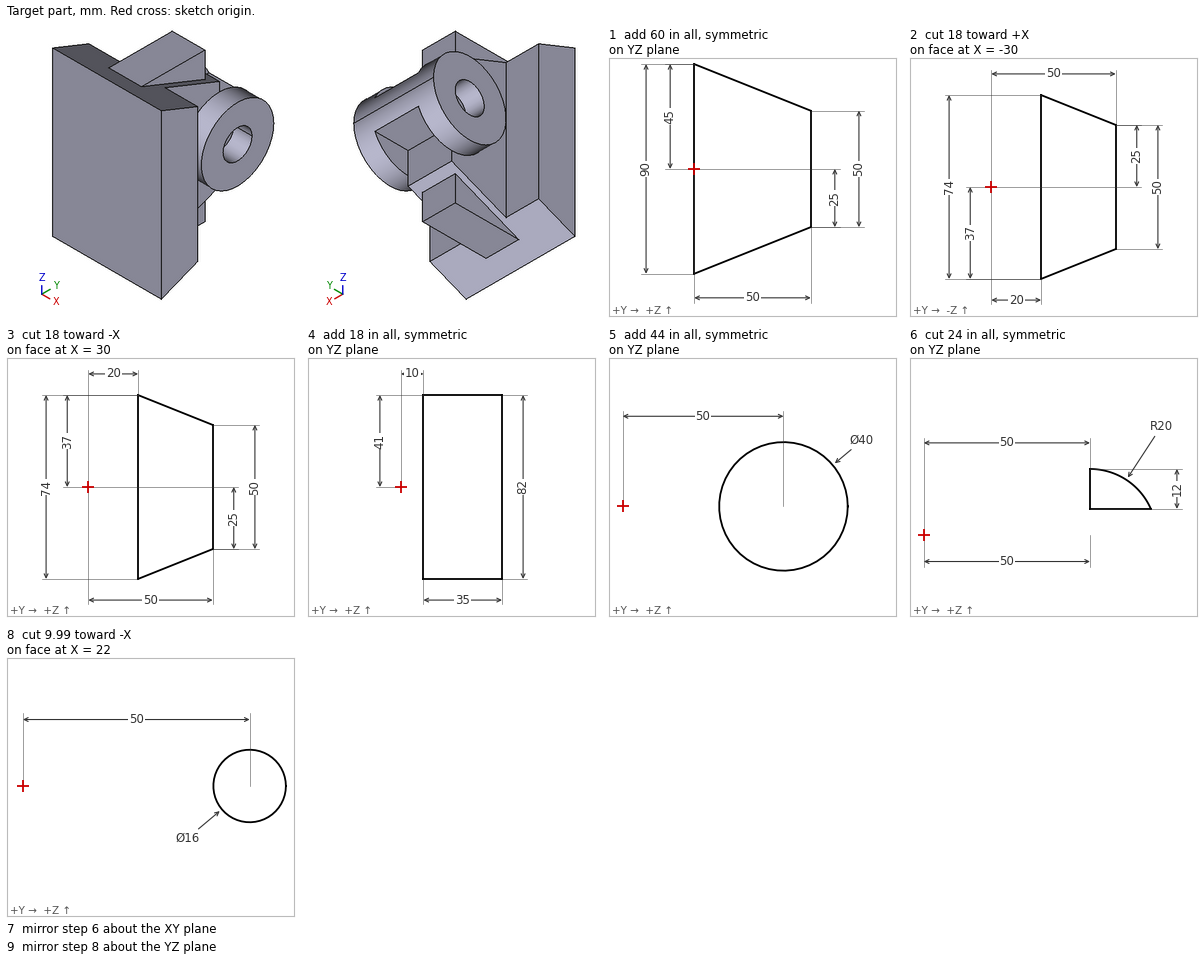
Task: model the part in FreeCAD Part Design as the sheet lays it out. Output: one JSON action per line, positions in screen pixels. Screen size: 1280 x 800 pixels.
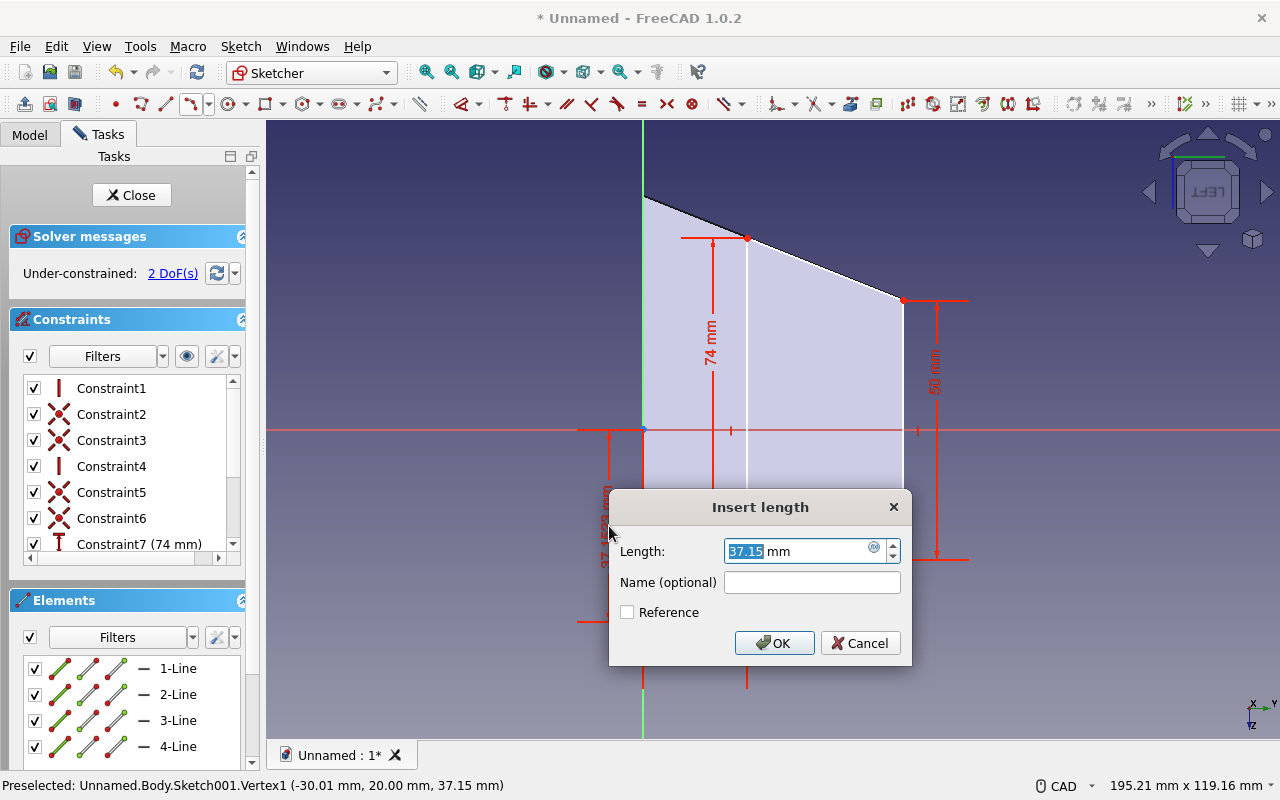
{"action": "type", "text": "37"}
{"action": "key", "text": "Return"}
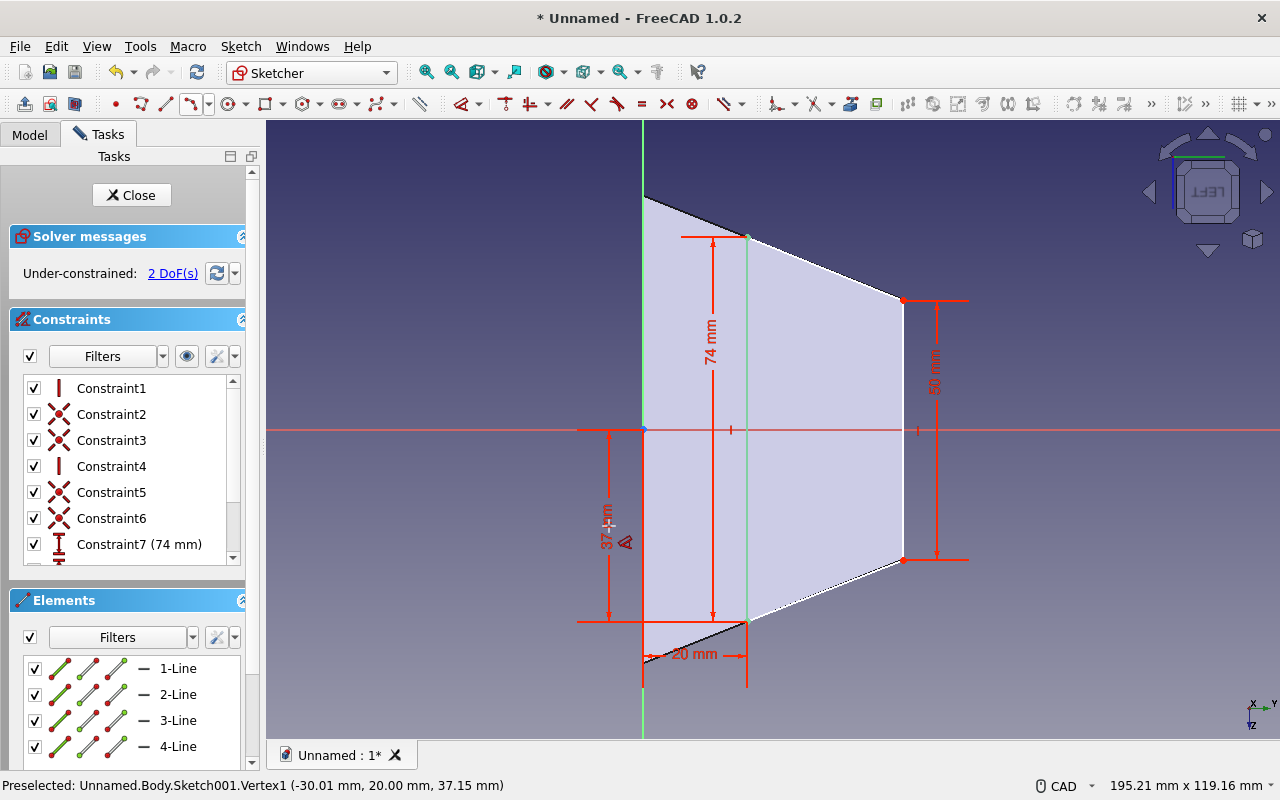
{"action": "left_click", "coordinate": [903, 301]}
{"action": "left_click", "coordinate": [773, 267]}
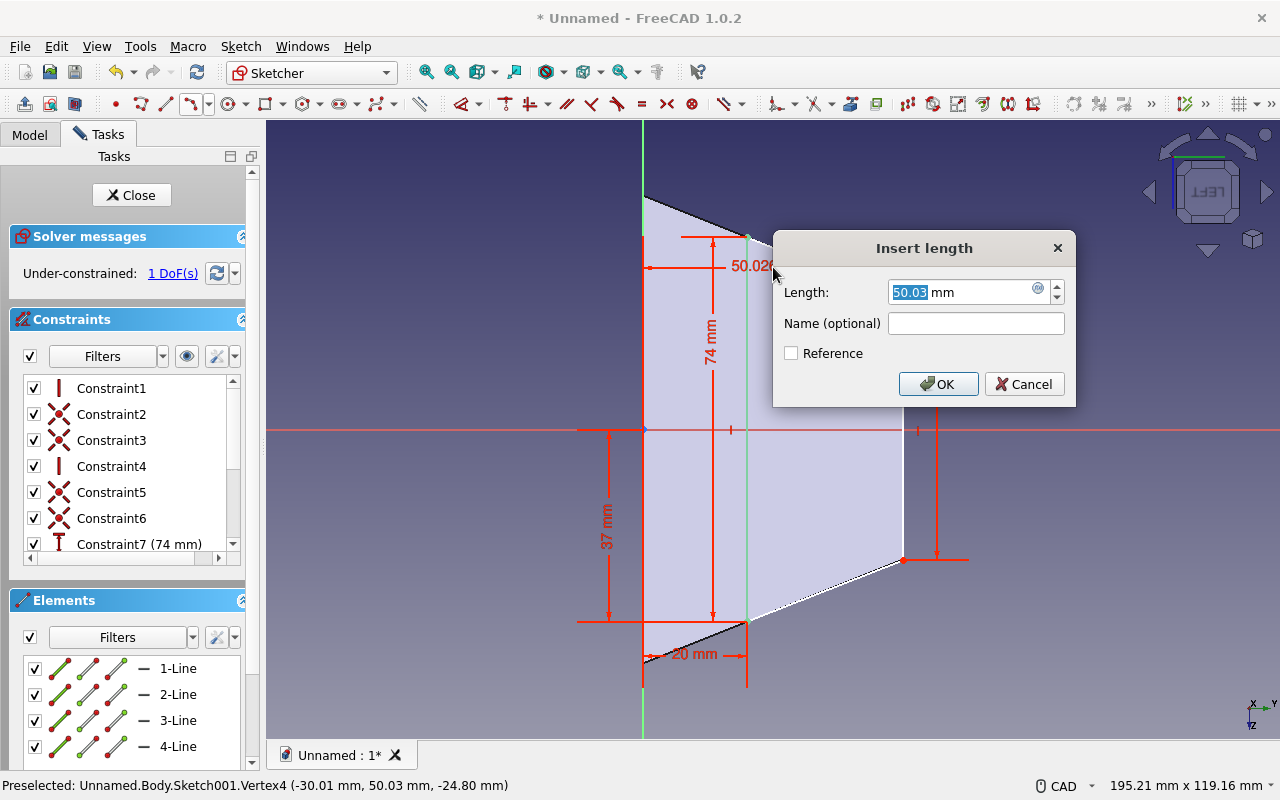
{"action": "type", "text": "50"}
{"action": "key", "text": "Return"}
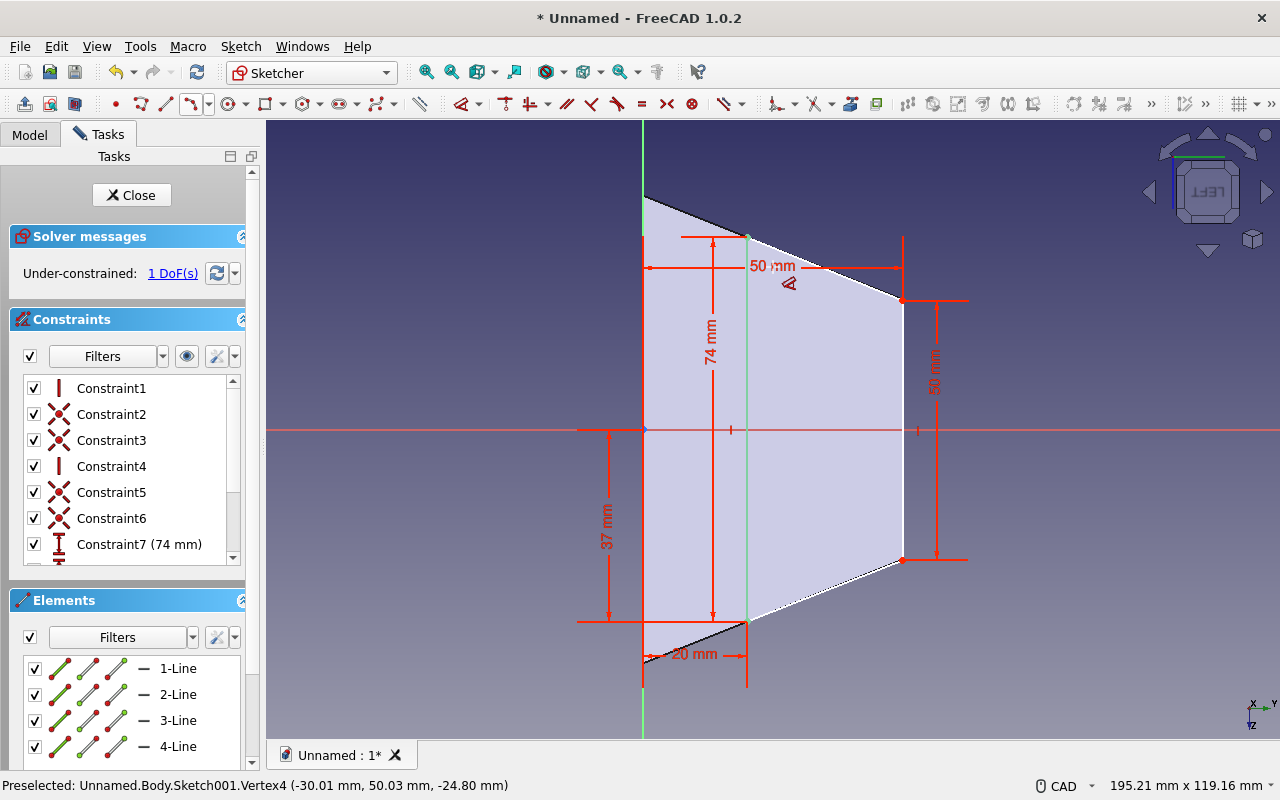
{"action": "left_click", "coordinate": [903, 301]}
{"action": "left_click", "coordinate": [937, 335]}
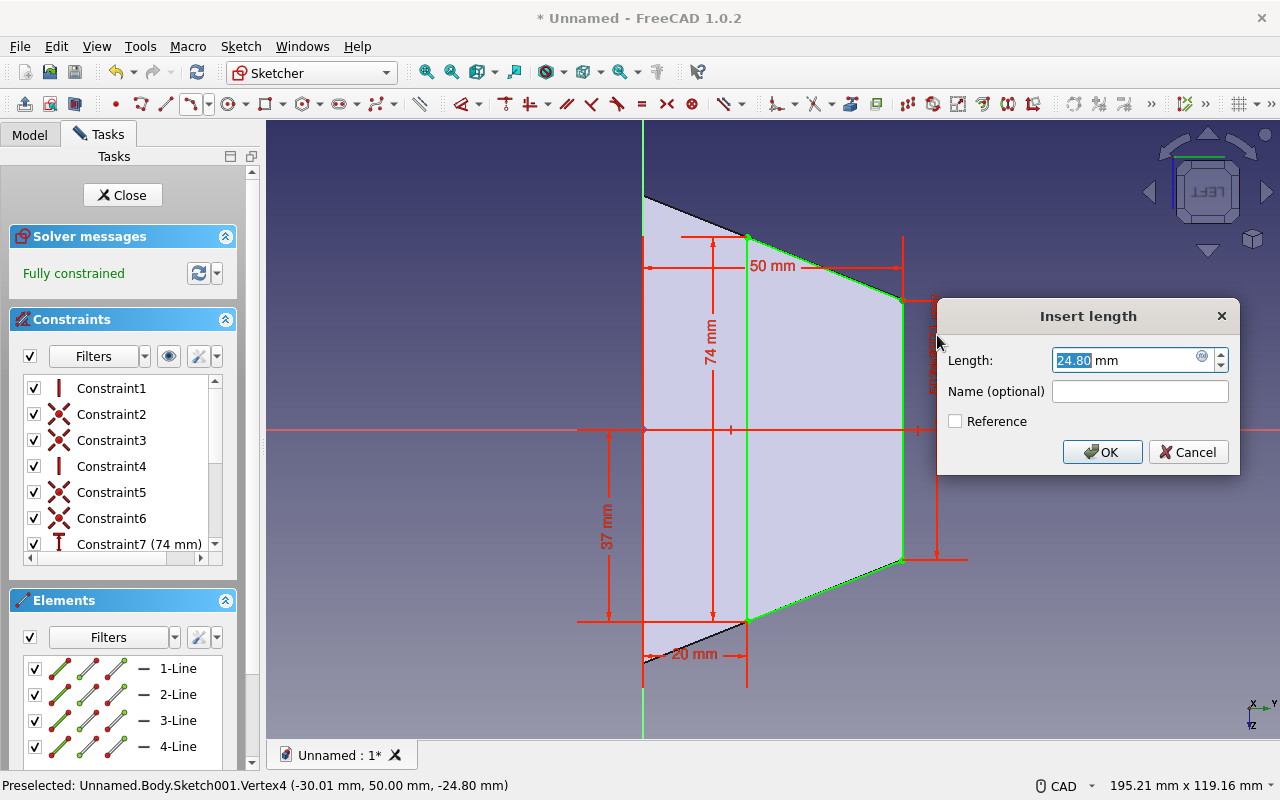
{"action": "type", "text": "25"}
{"action": "key", "text": "Return"}
{"action": "key", "text": "Escape"}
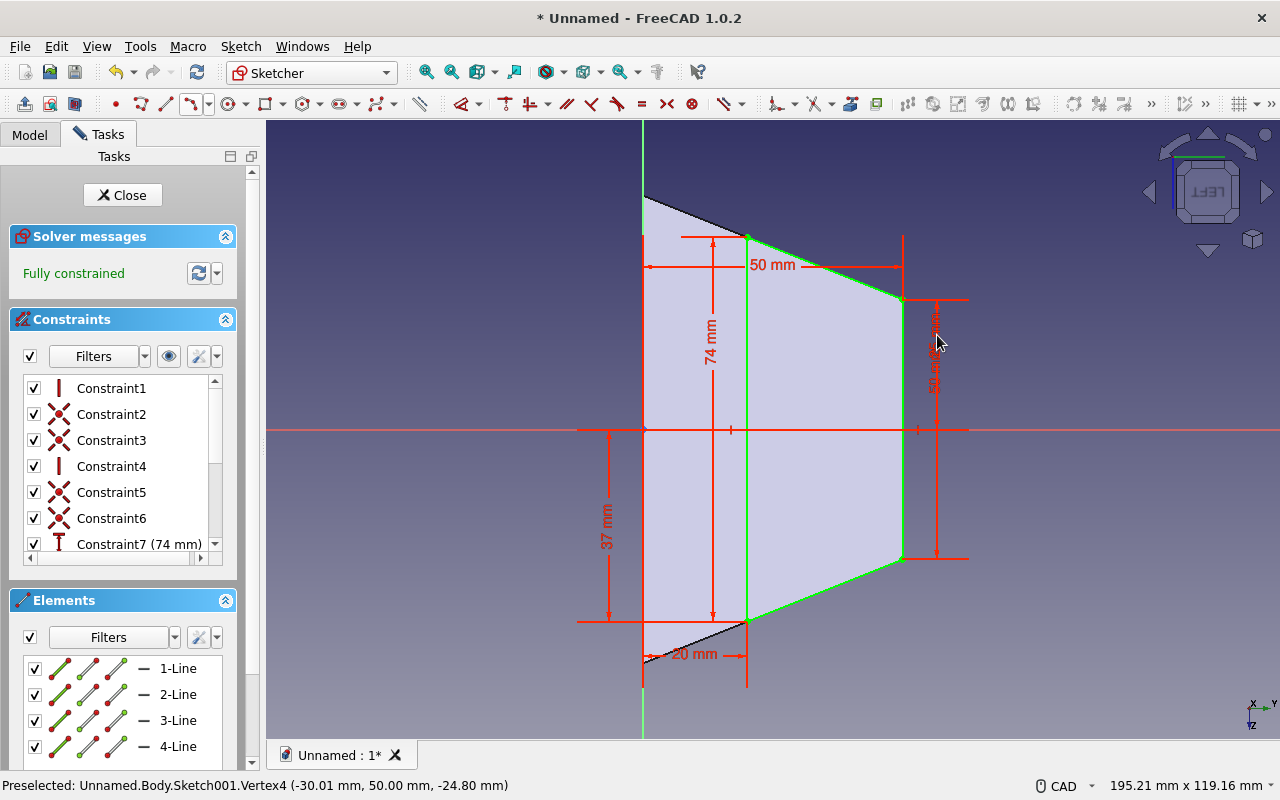
{"action": "left_click", "coordinate": [123, 195]}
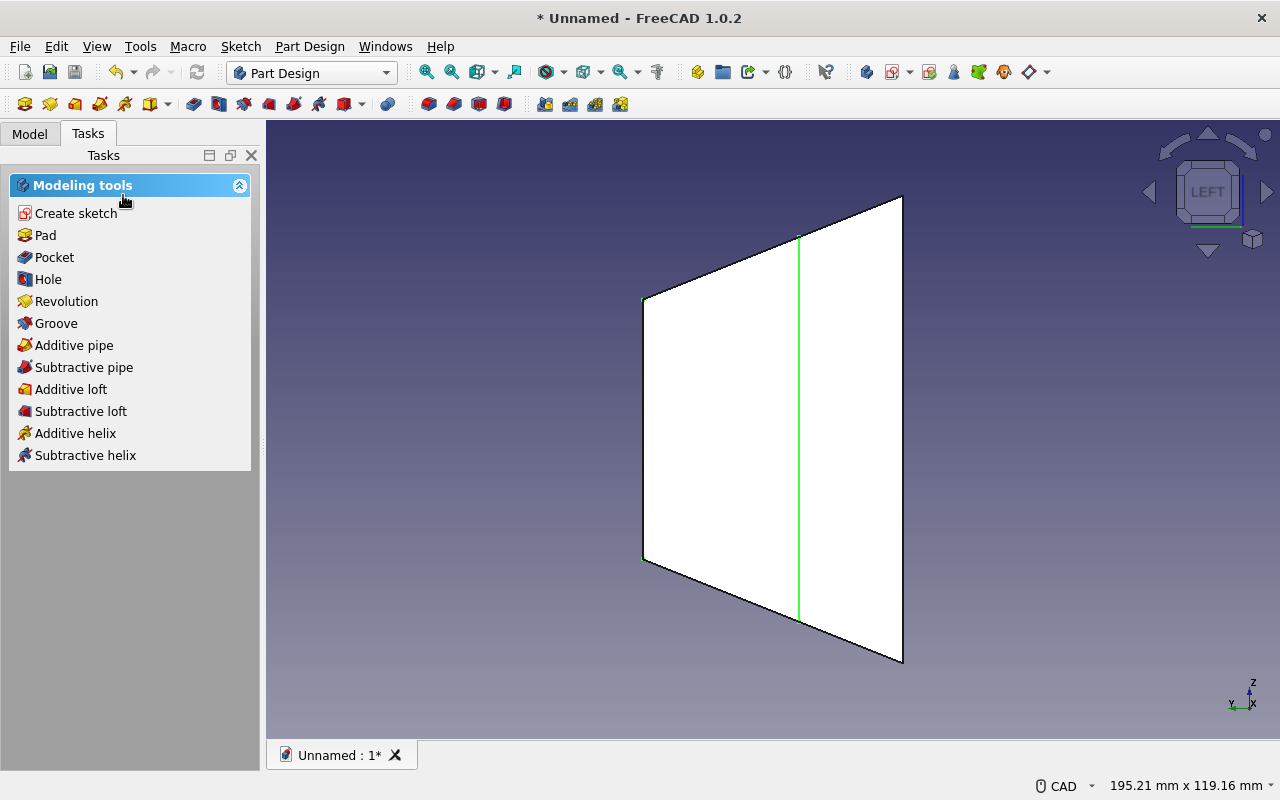
{"action": "left_click", "coordinate": [194, 104]}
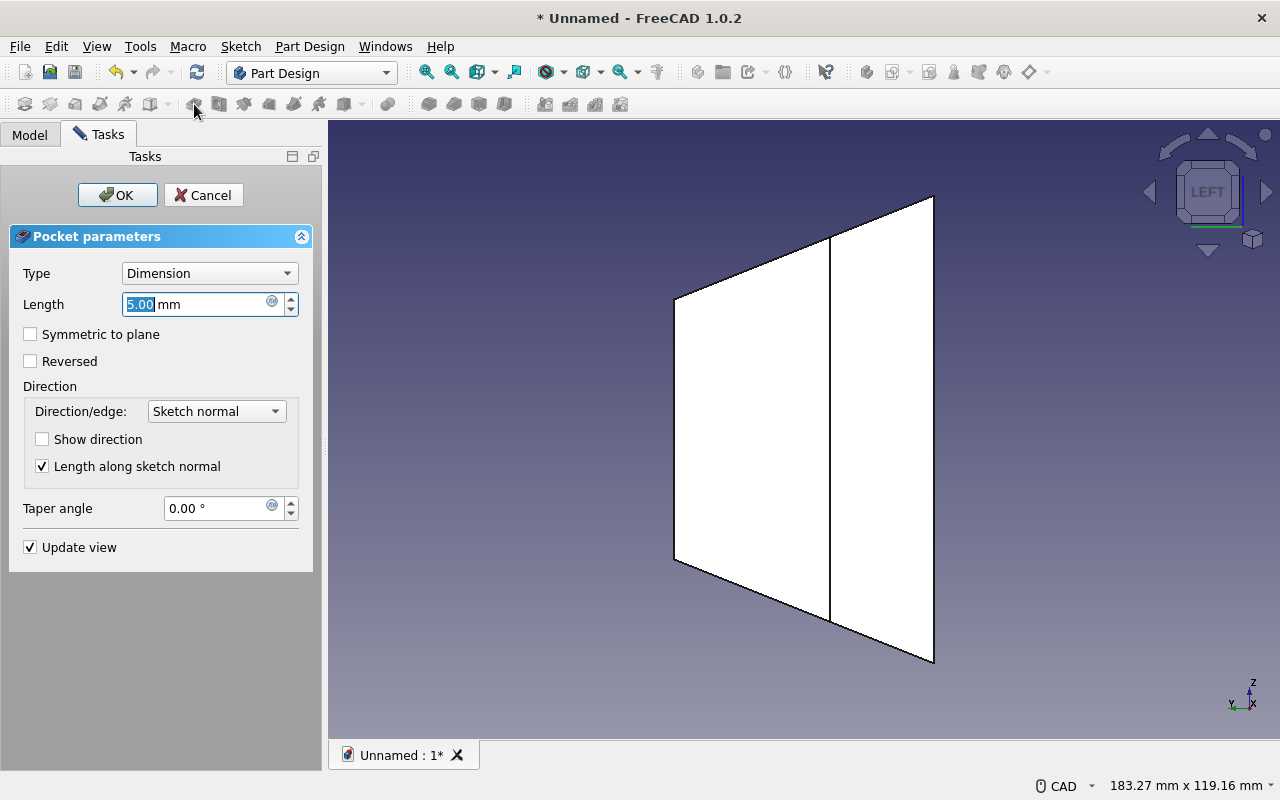
{"action": "type", "text": "18"}
{"action": "key", "text": "Tab"}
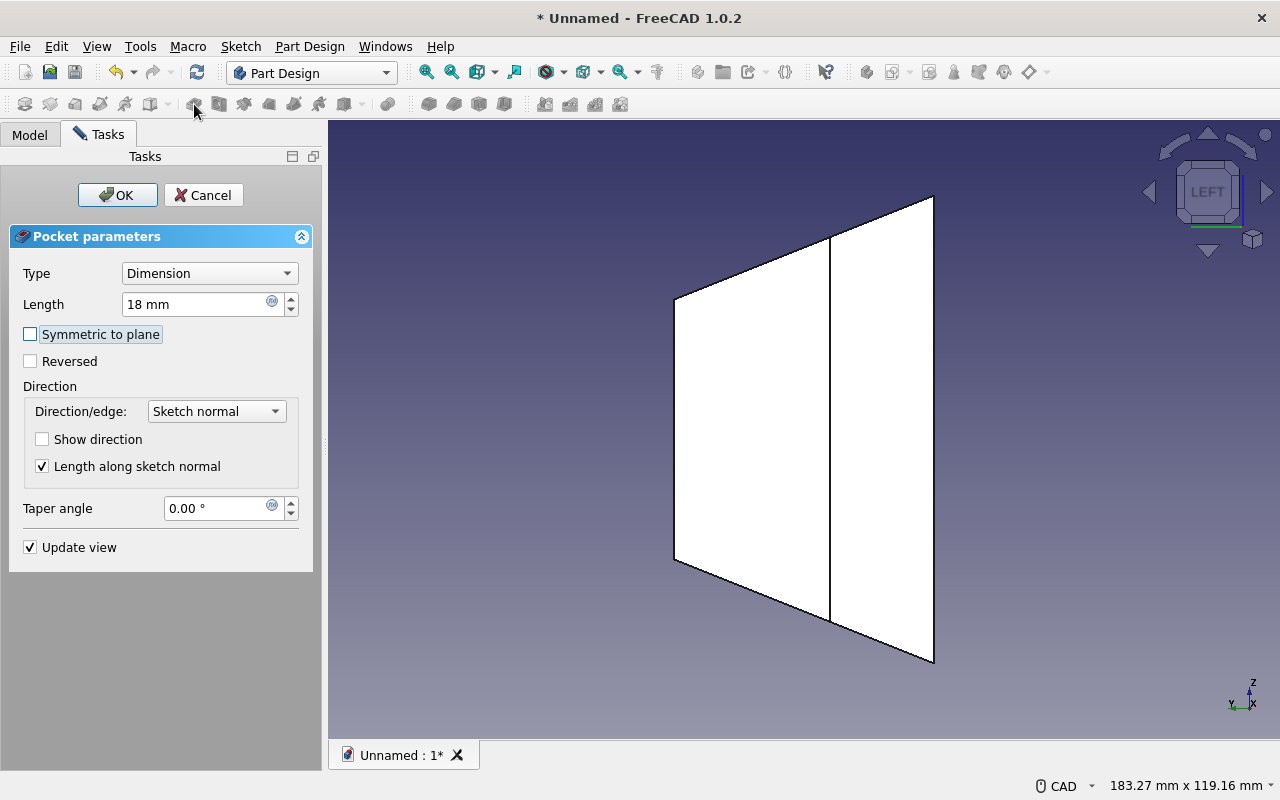
{"action": "left_click", "coordinate": [118, 195]}